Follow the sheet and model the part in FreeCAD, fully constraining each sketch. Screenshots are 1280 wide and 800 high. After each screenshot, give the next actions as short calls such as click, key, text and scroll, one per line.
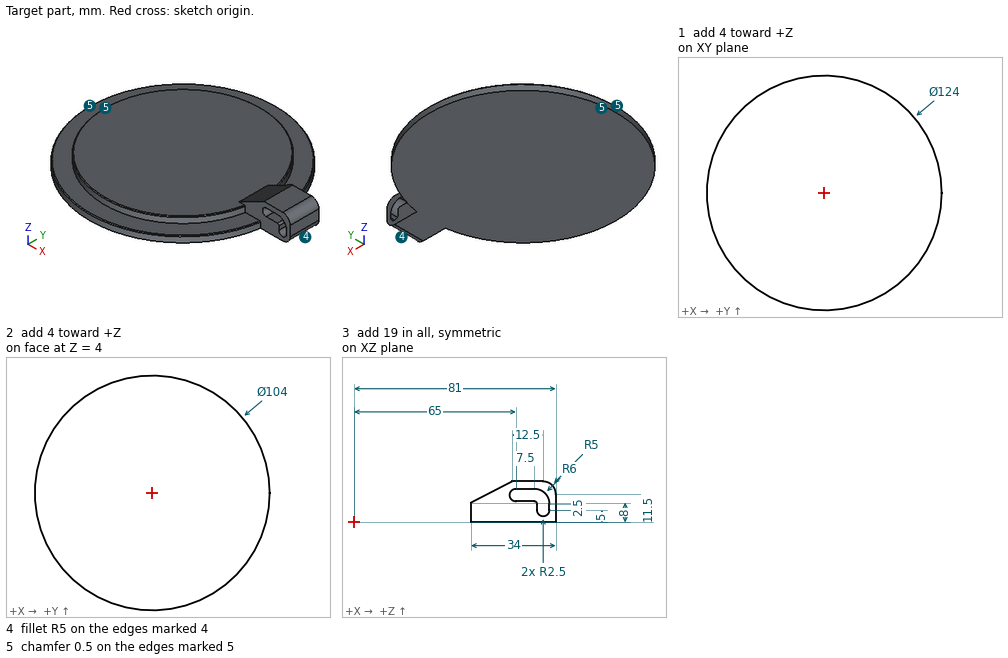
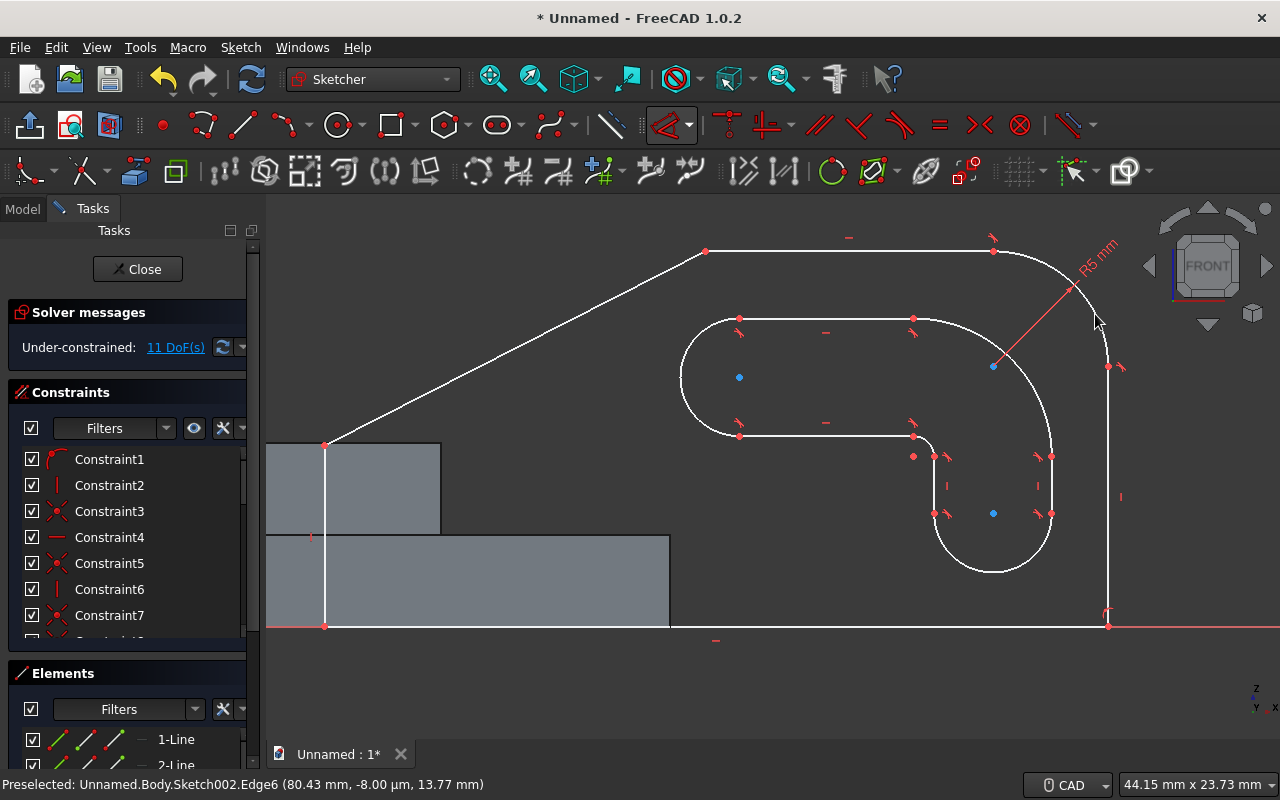
click(1037, 394)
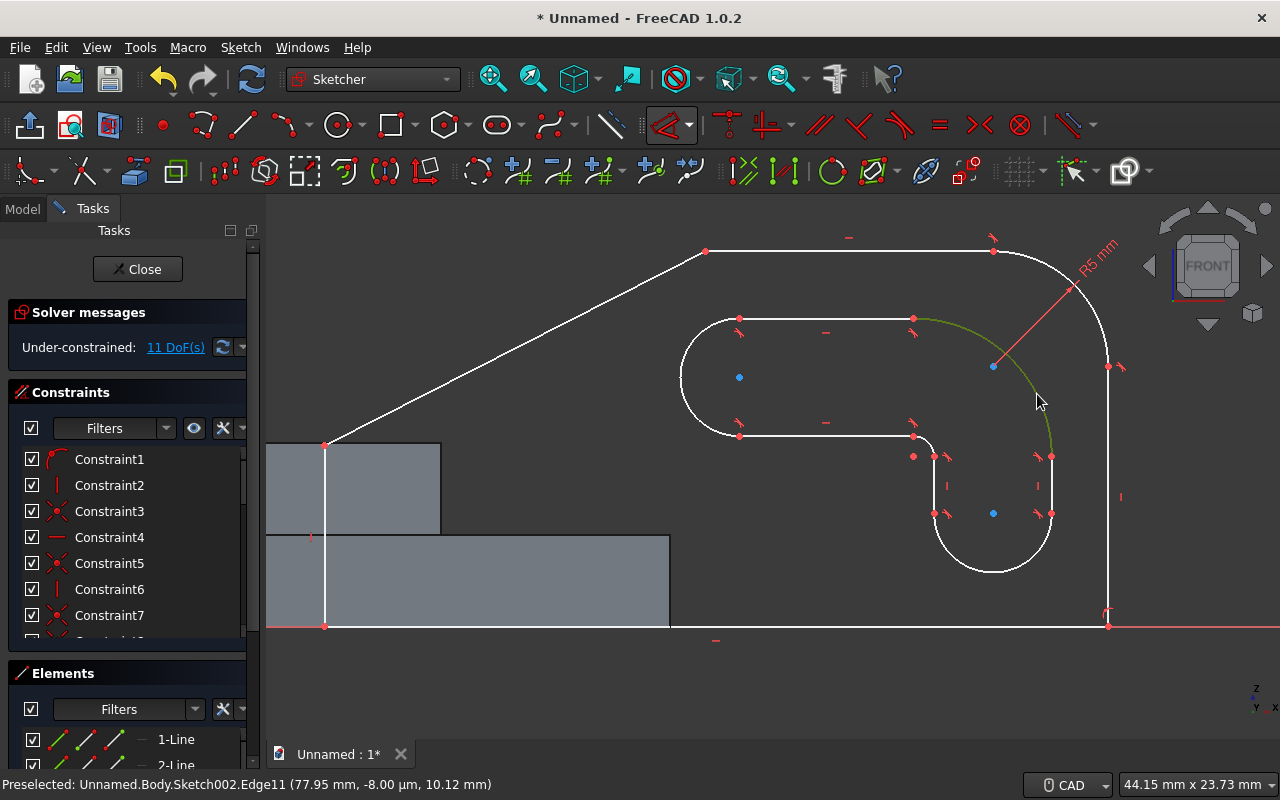
key(k)
key(r)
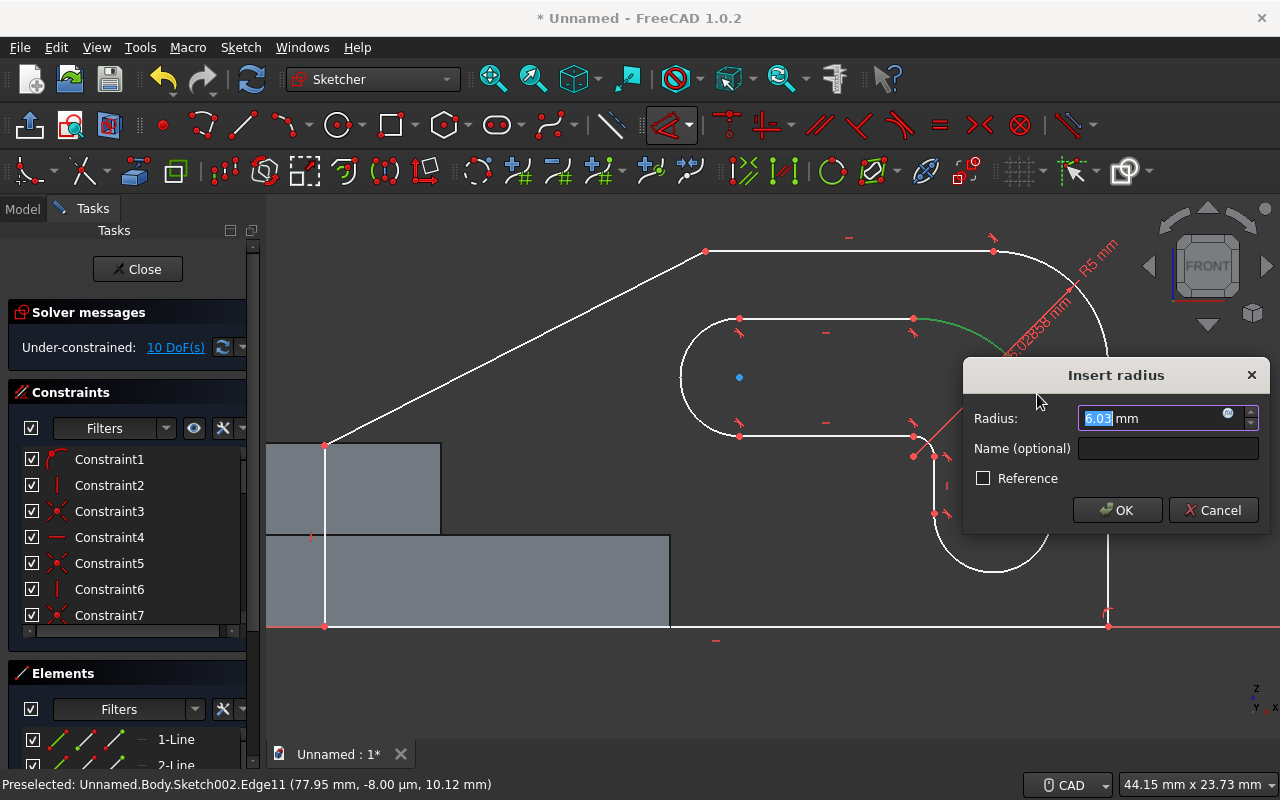
text(6)
key(Return)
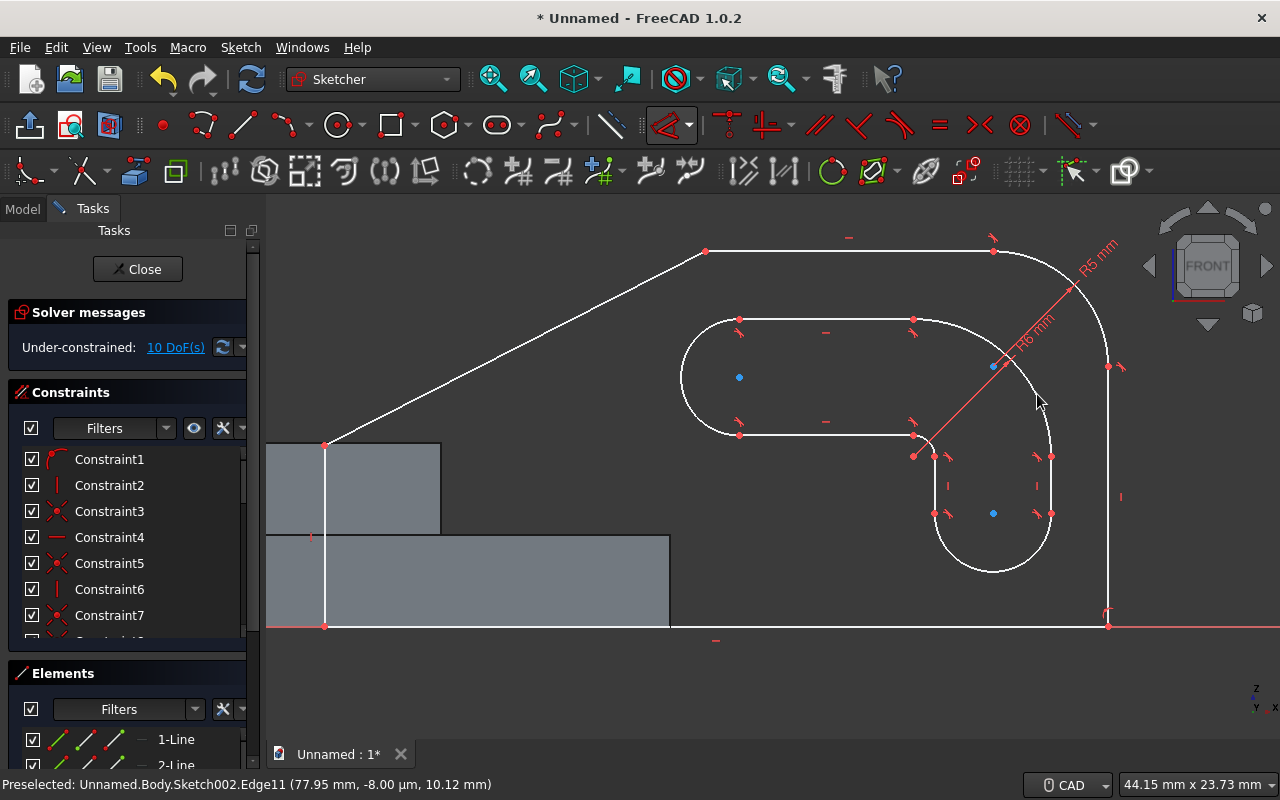
click(692, 343)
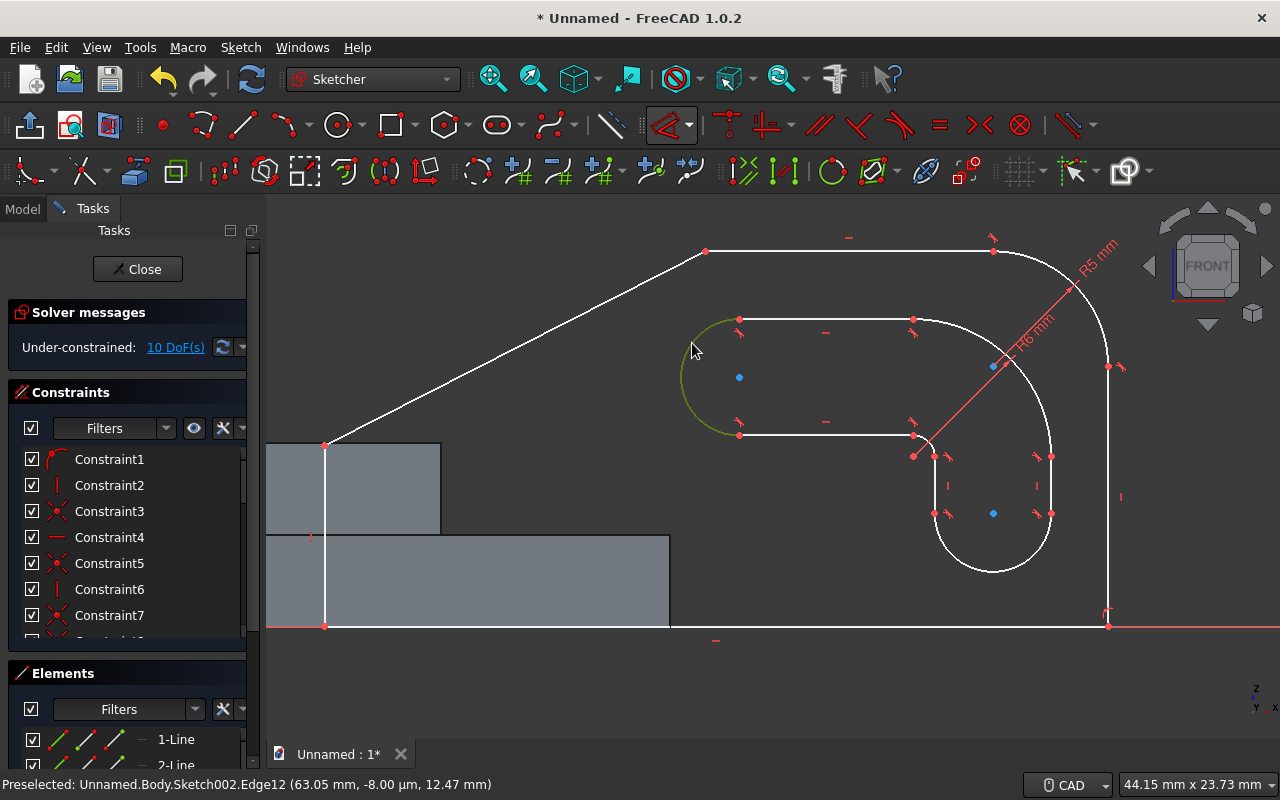
key(k)
key(r)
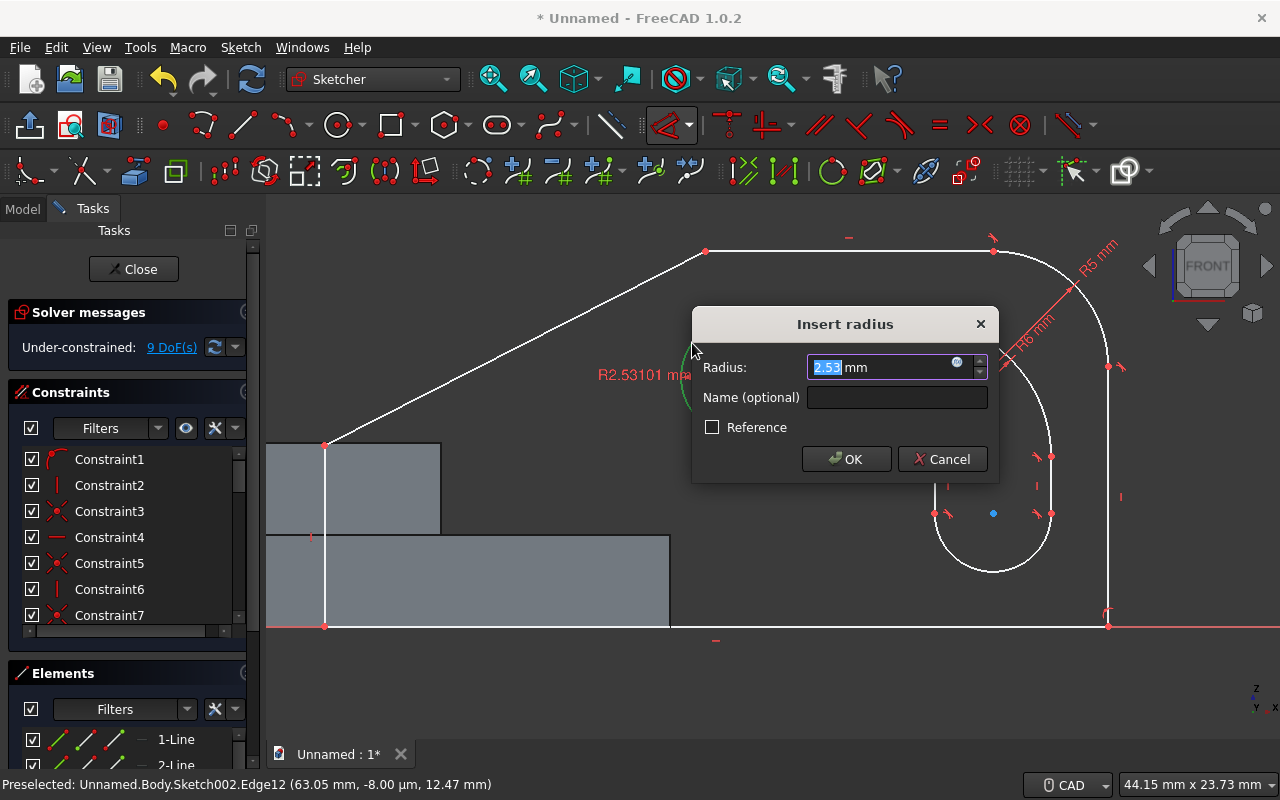
text(2.5)
key(Return)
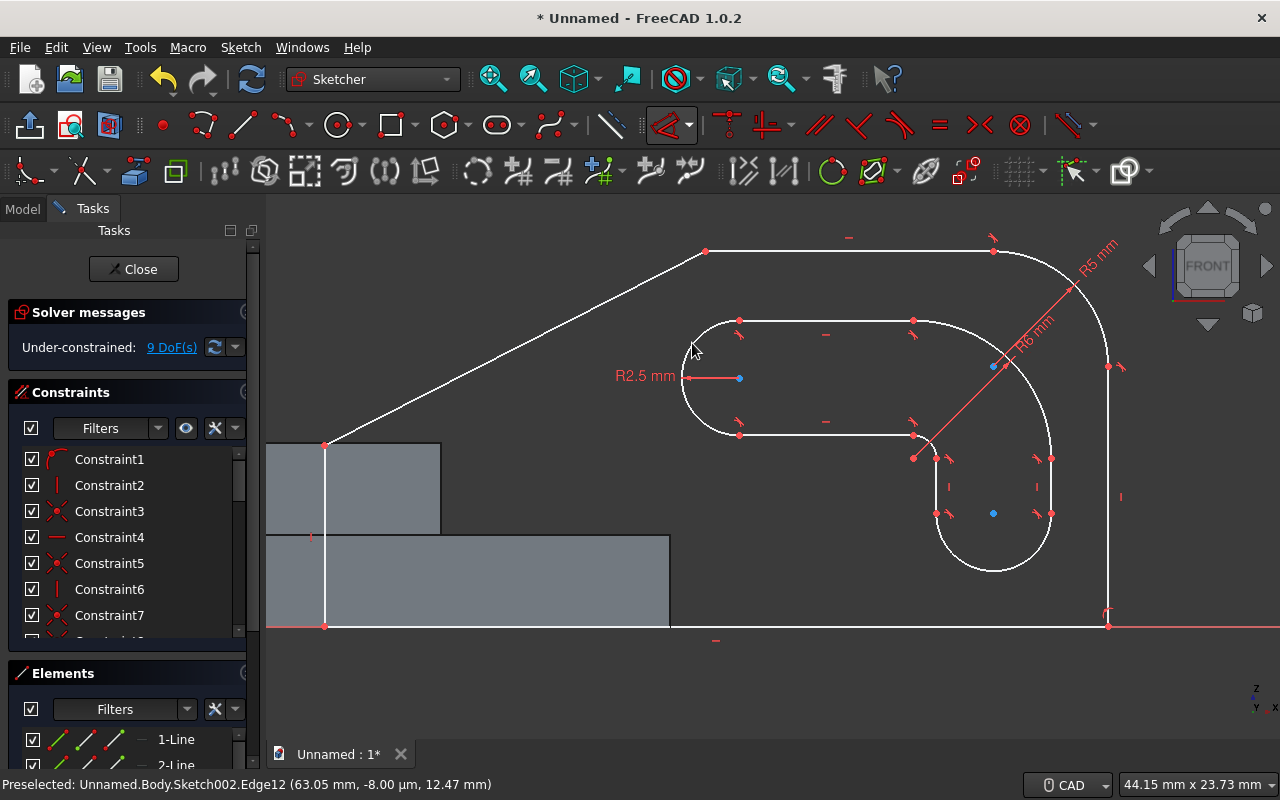
click(325, 572)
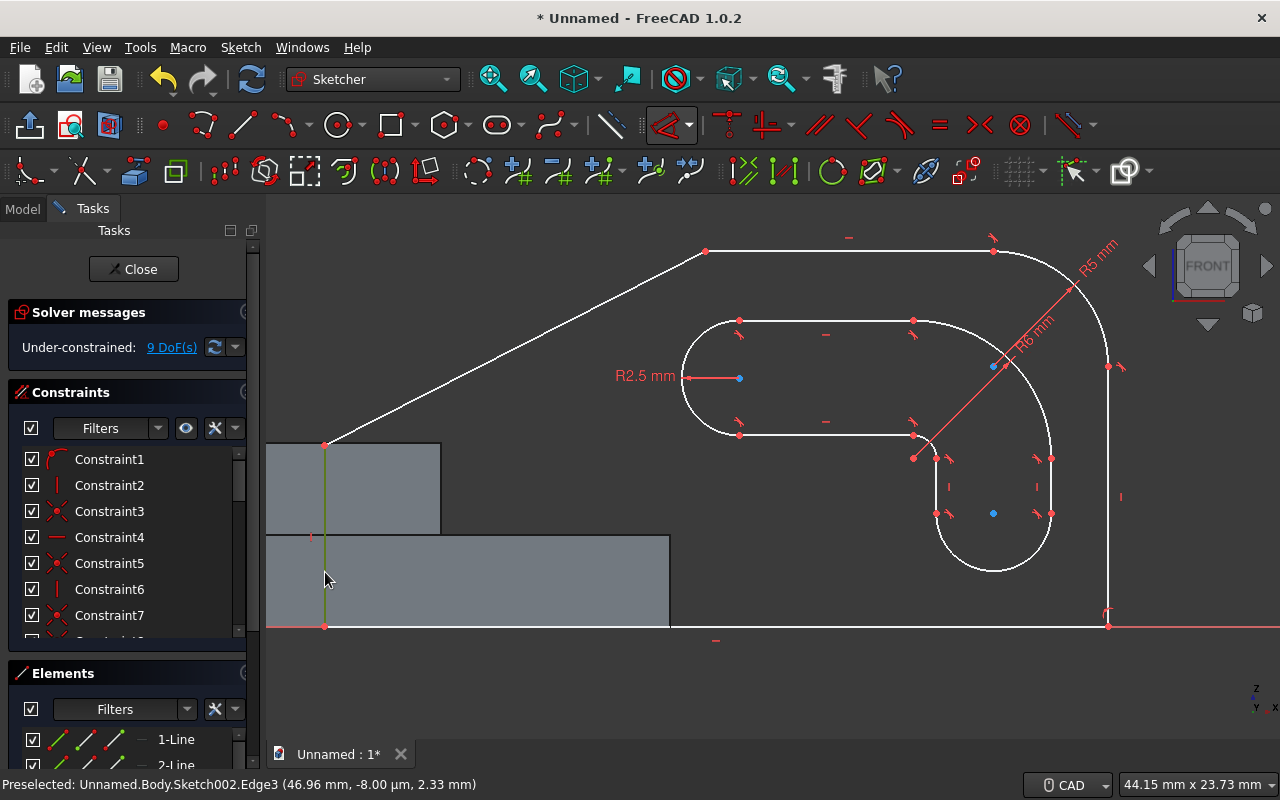
key(i)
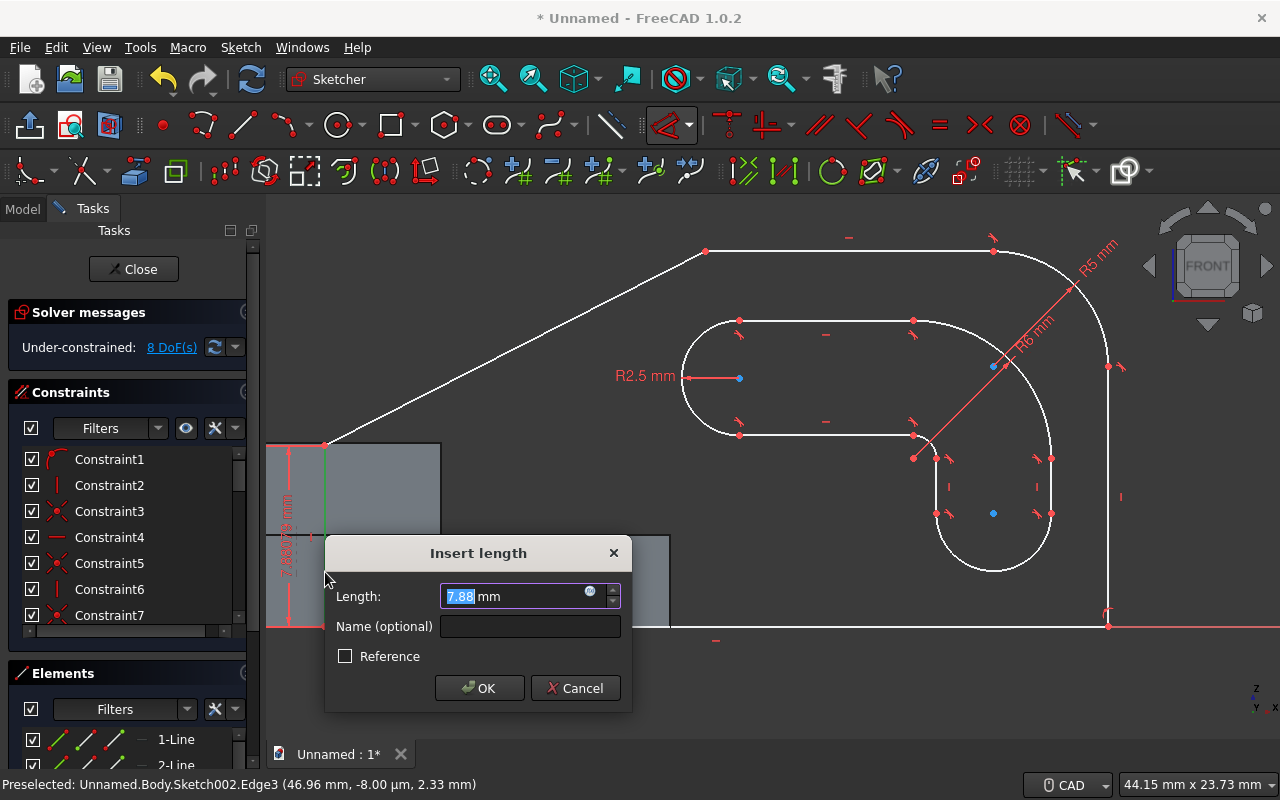
text(8)
key(Return)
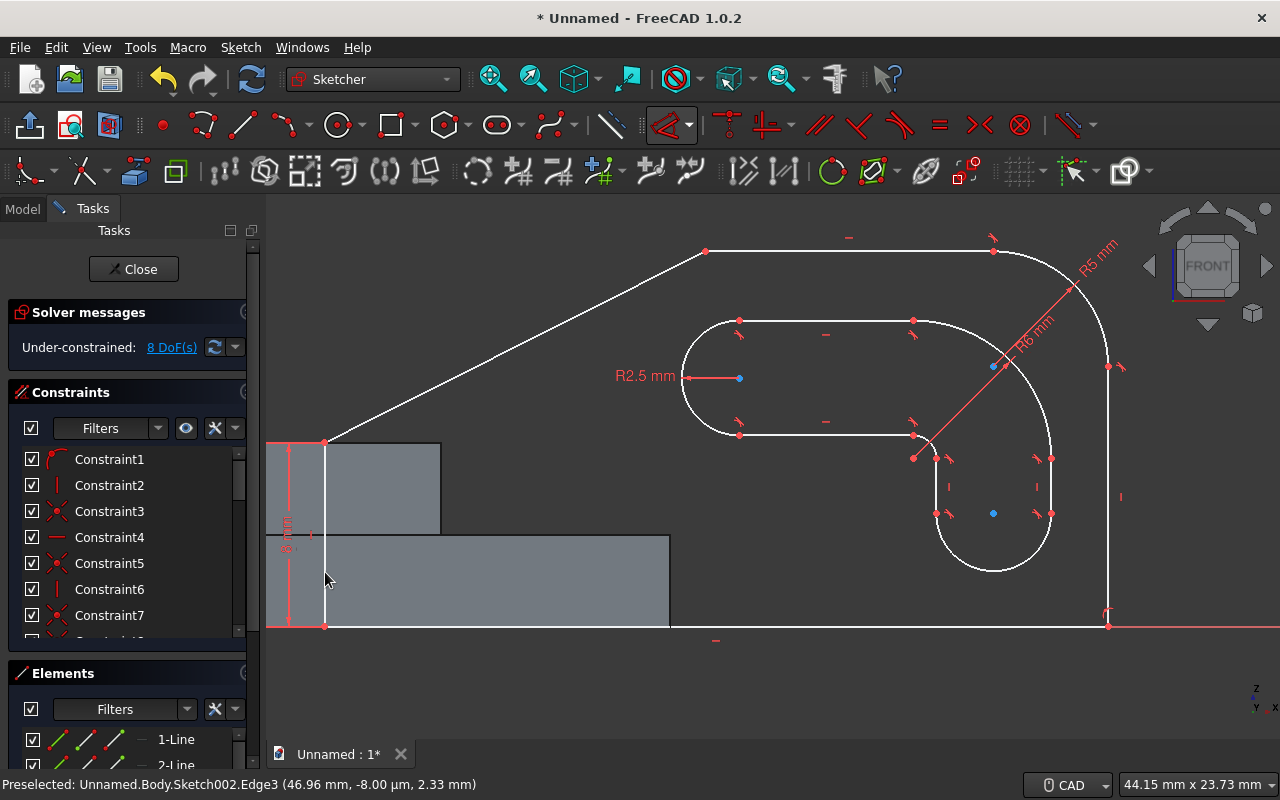
click(873, 627)